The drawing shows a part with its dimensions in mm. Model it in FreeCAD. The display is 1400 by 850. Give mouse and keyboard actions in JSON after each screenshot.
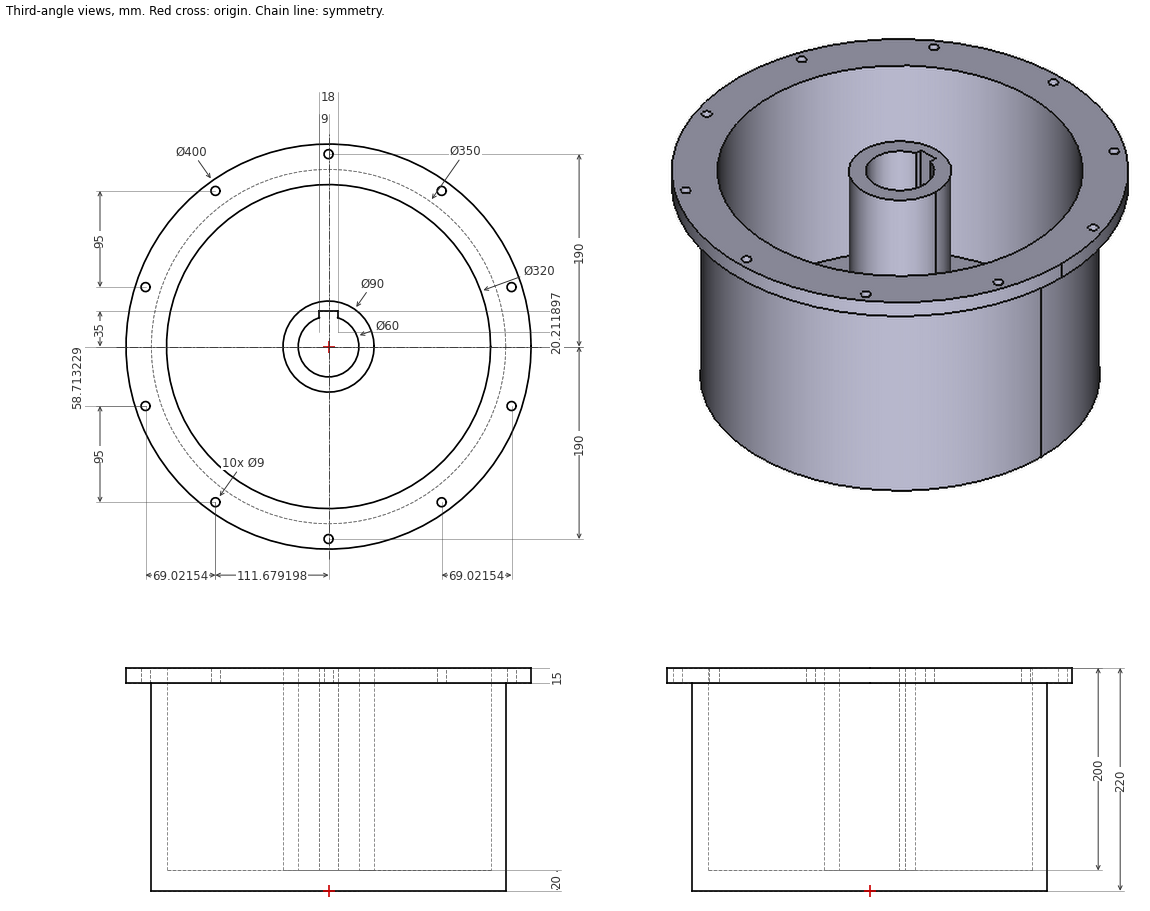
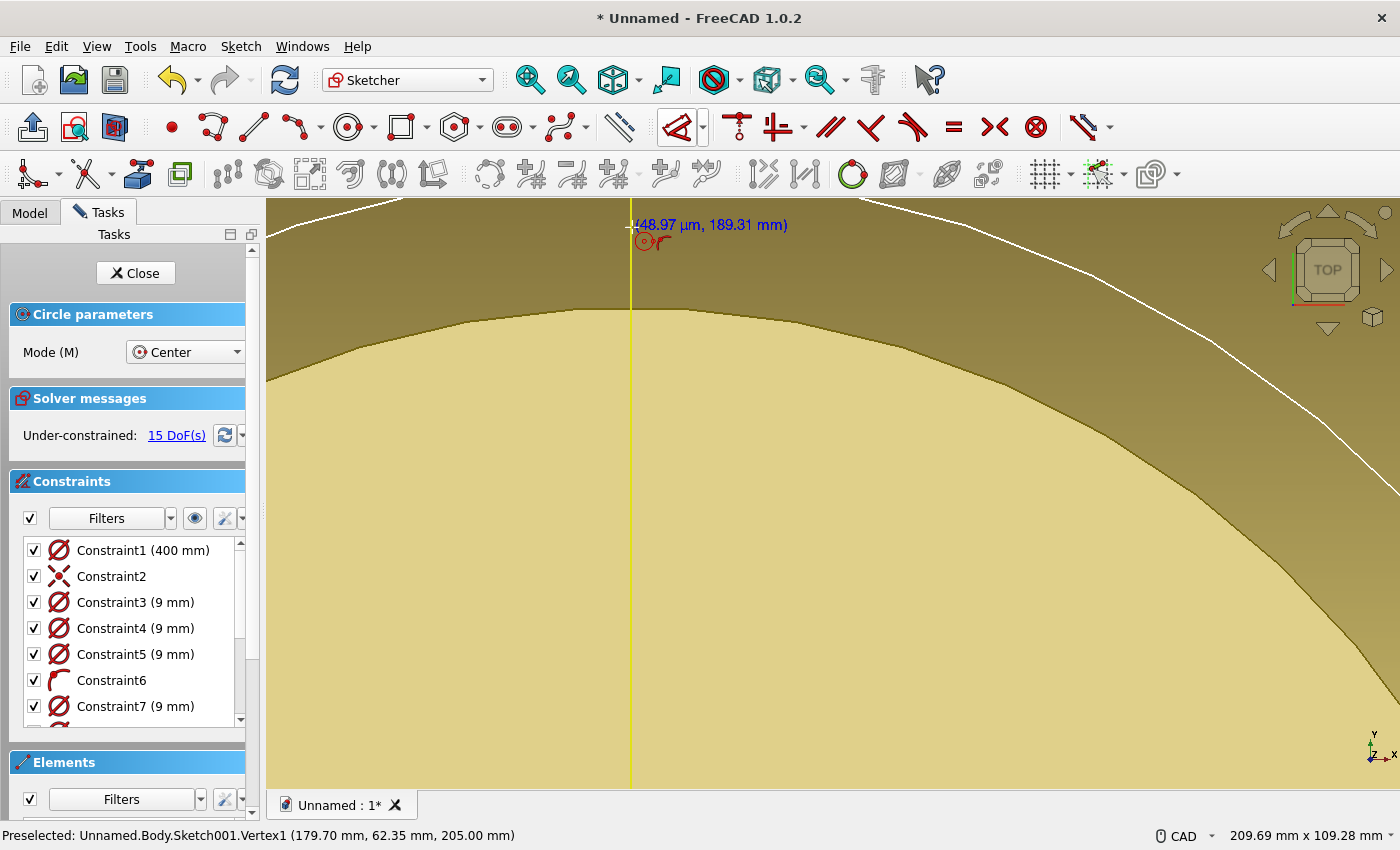
{"action": "scroll", "coordinate": [791, 343], "scroll_direction": "down", "scroll_amount": 9}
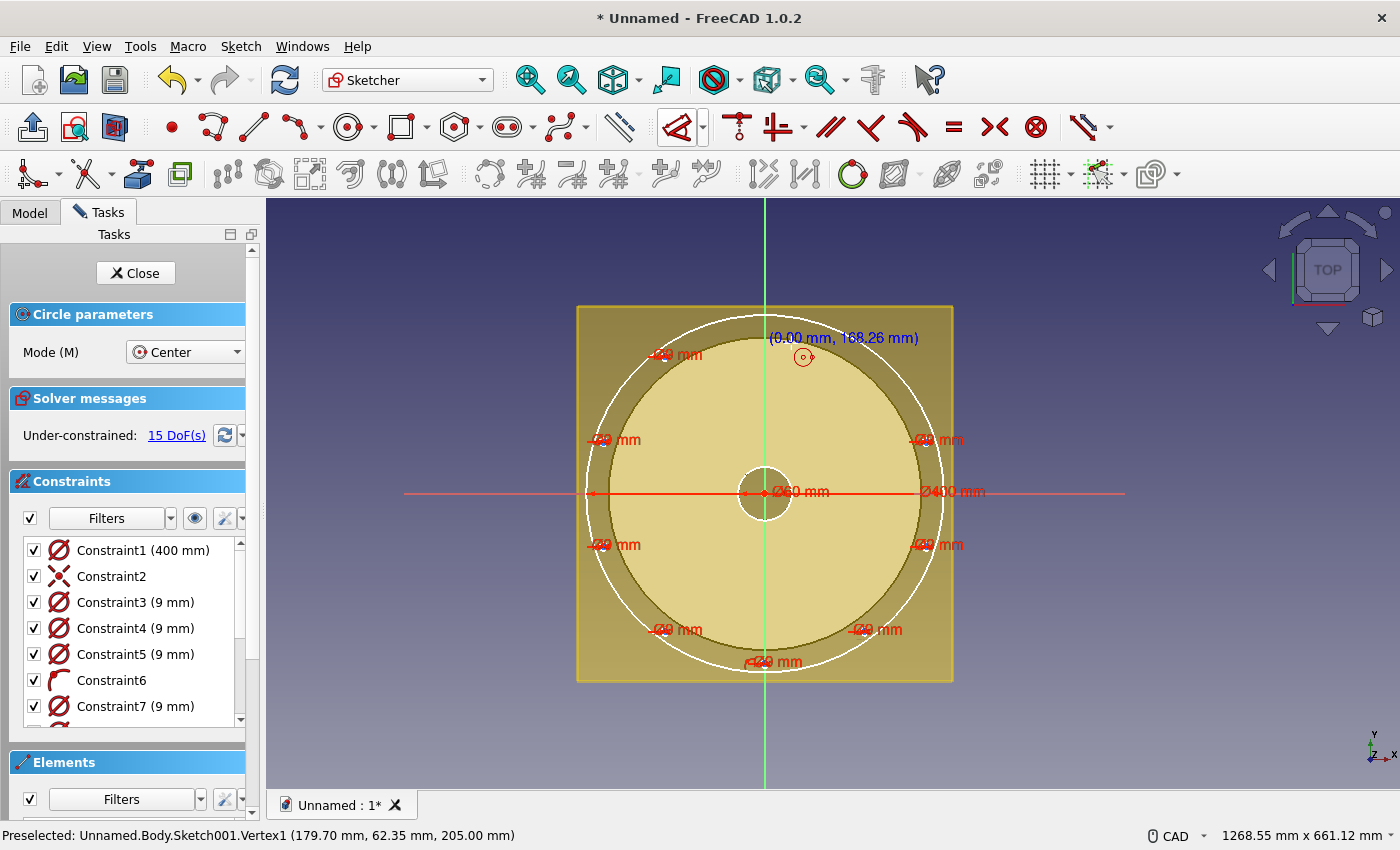
{"action": "scroll", "coordinate": [765, 324], "scroll_direction": "up", "scroll_amount": 3}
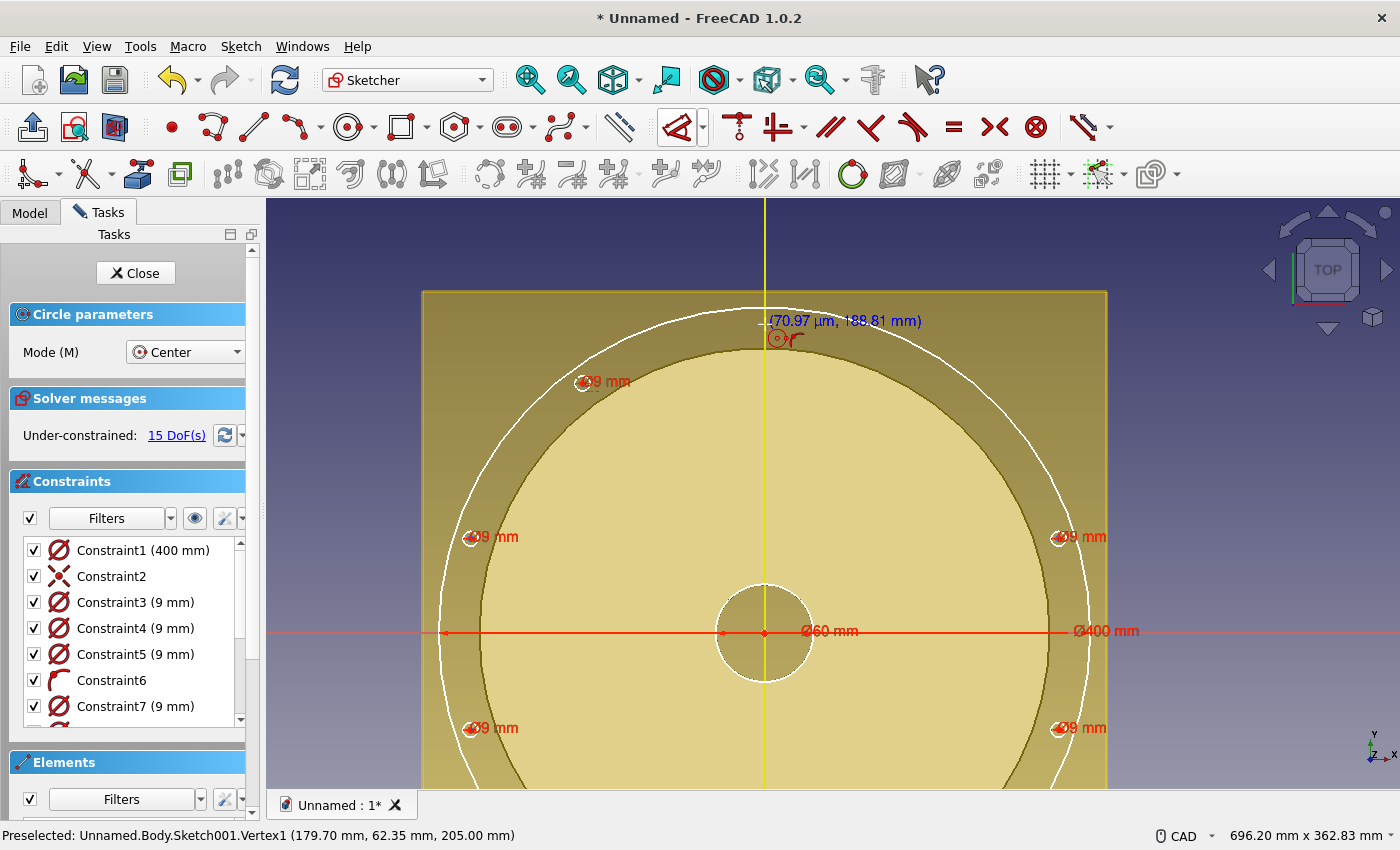
{"action": "left_click", "coordinate": [765, 324]}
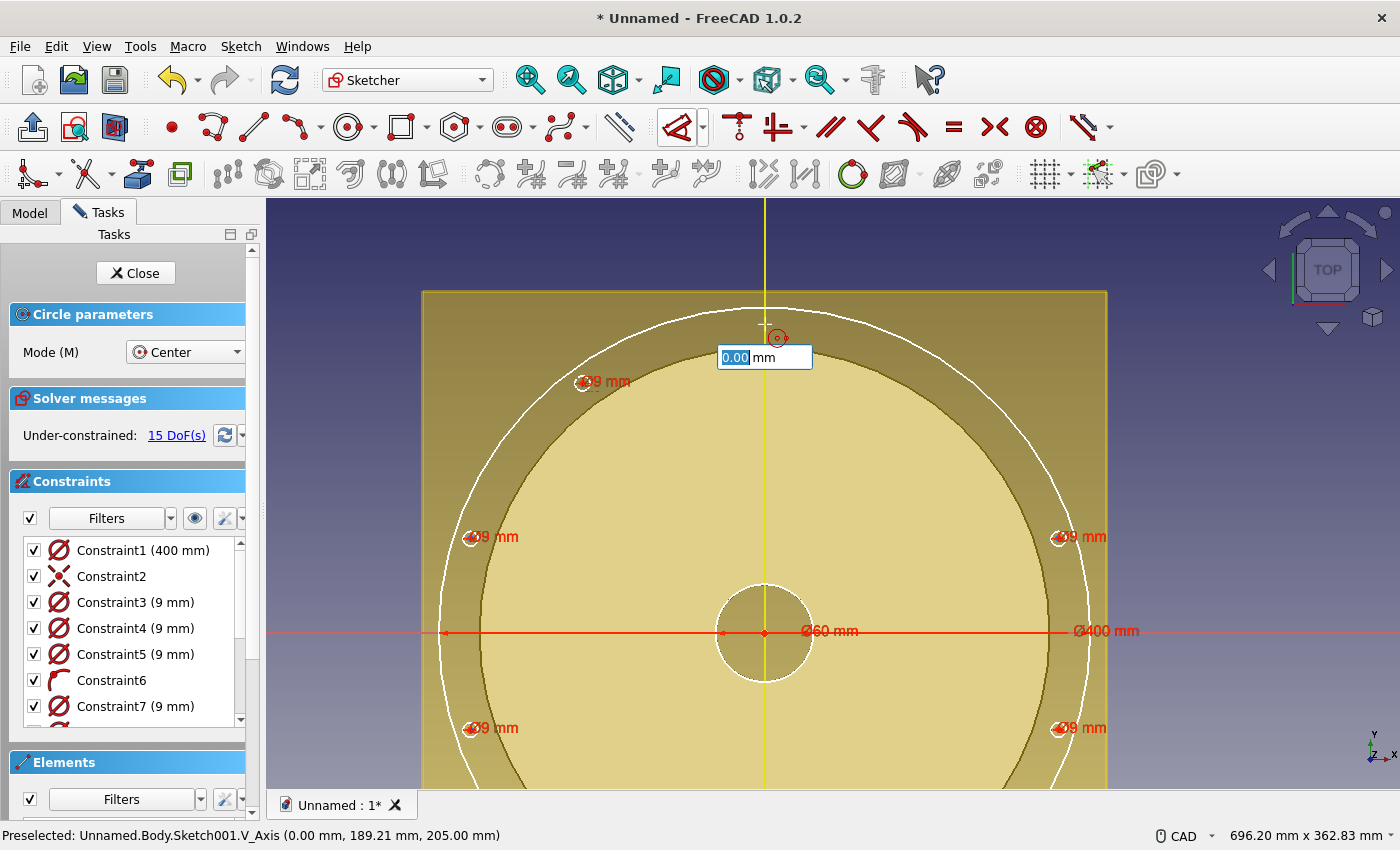
{"action": "scroll", "coordinate": [771, 321], "scroll_direction": "up", "scroll_amount": 5}
{"action": "mouse_move", "coordinate": [771, 321]}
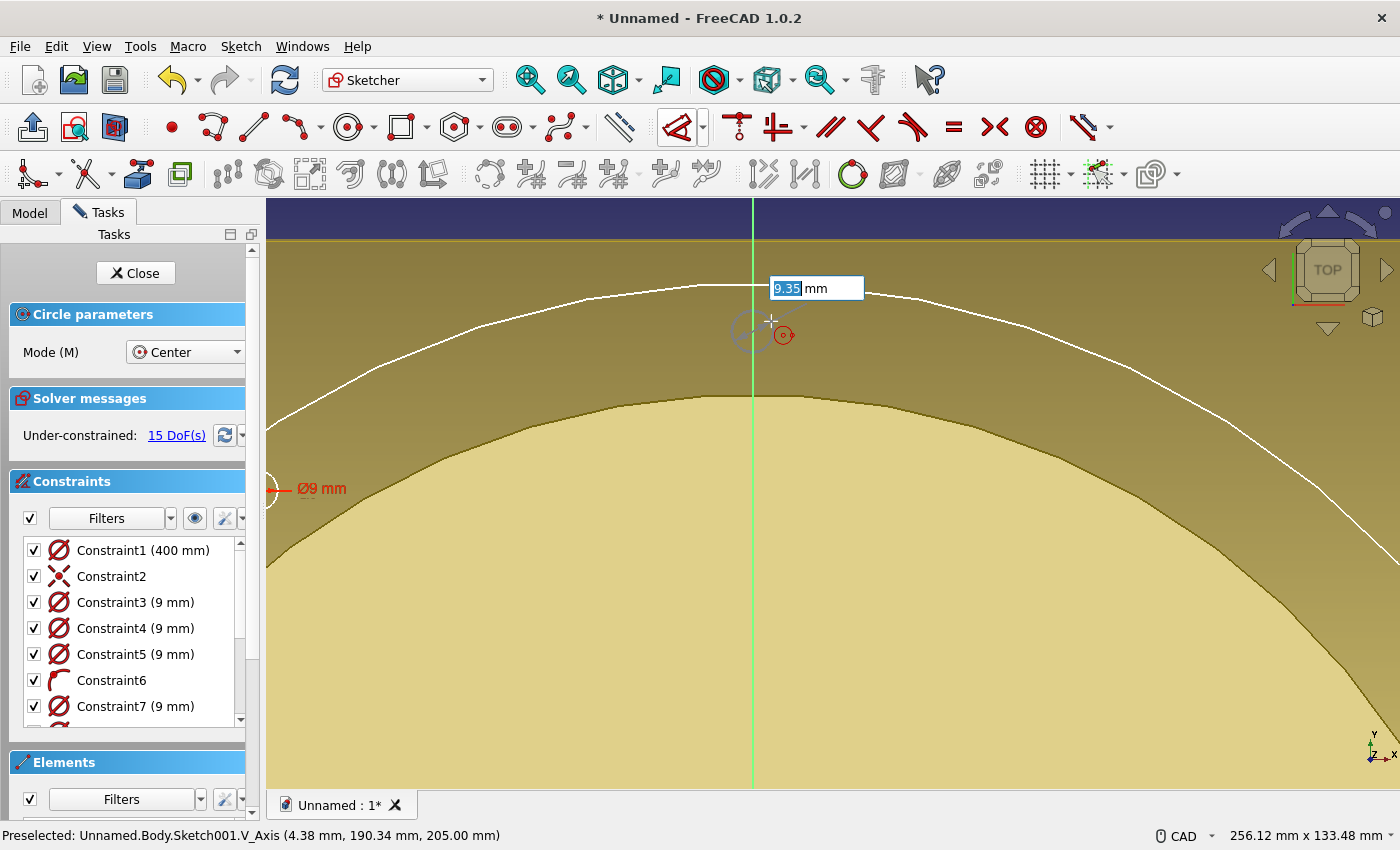
{"action": "type", "text": "9"}
{"action": "key", "text": "Return"}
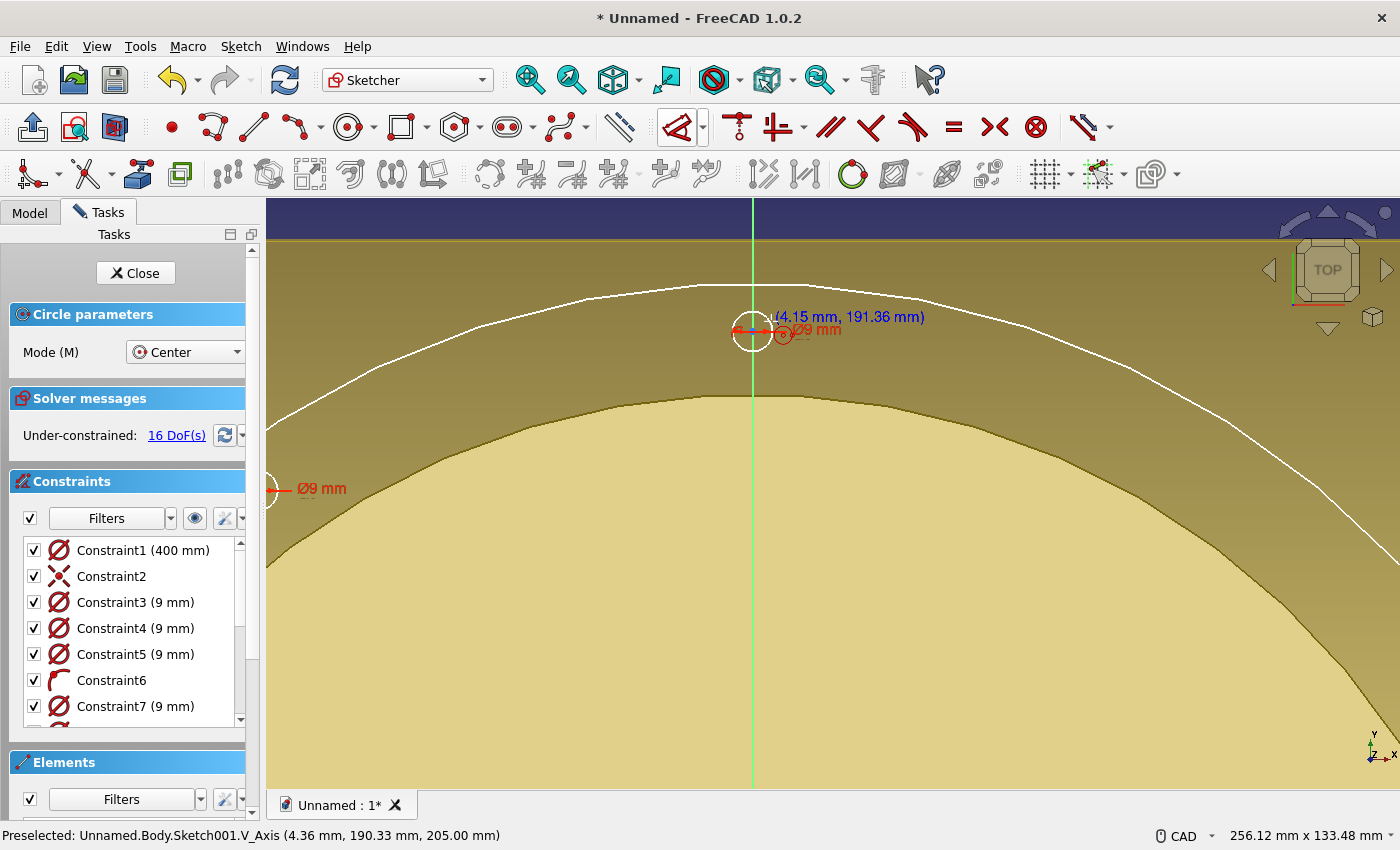
{"action": "scroll", "coordinate": [768, 323], "scroll_direction": "down", "scroll_amount": 8}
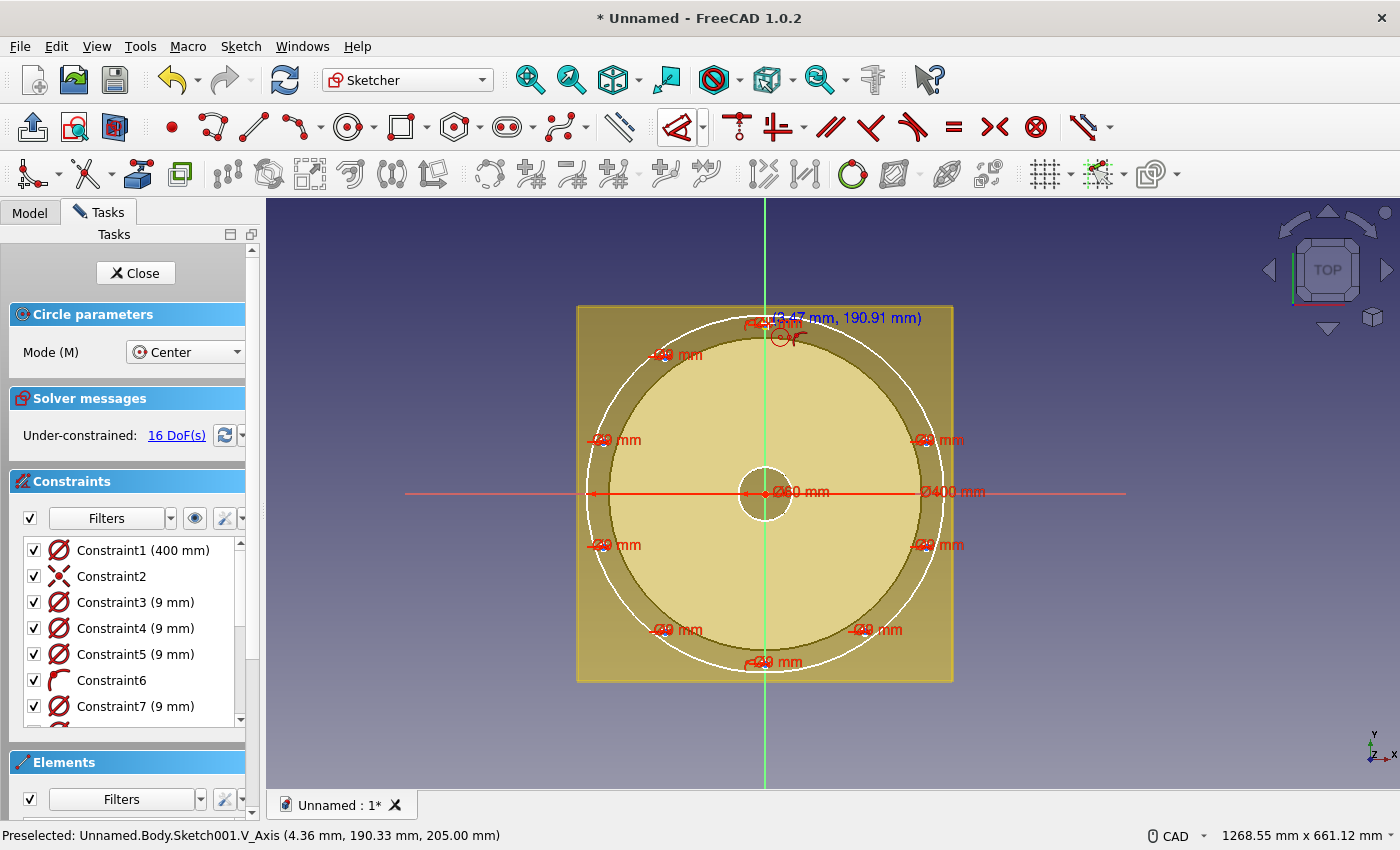
{"action": "scroll", "coordinate": [865, 357], "scroll_direction": "up", "scroll_amount": 9}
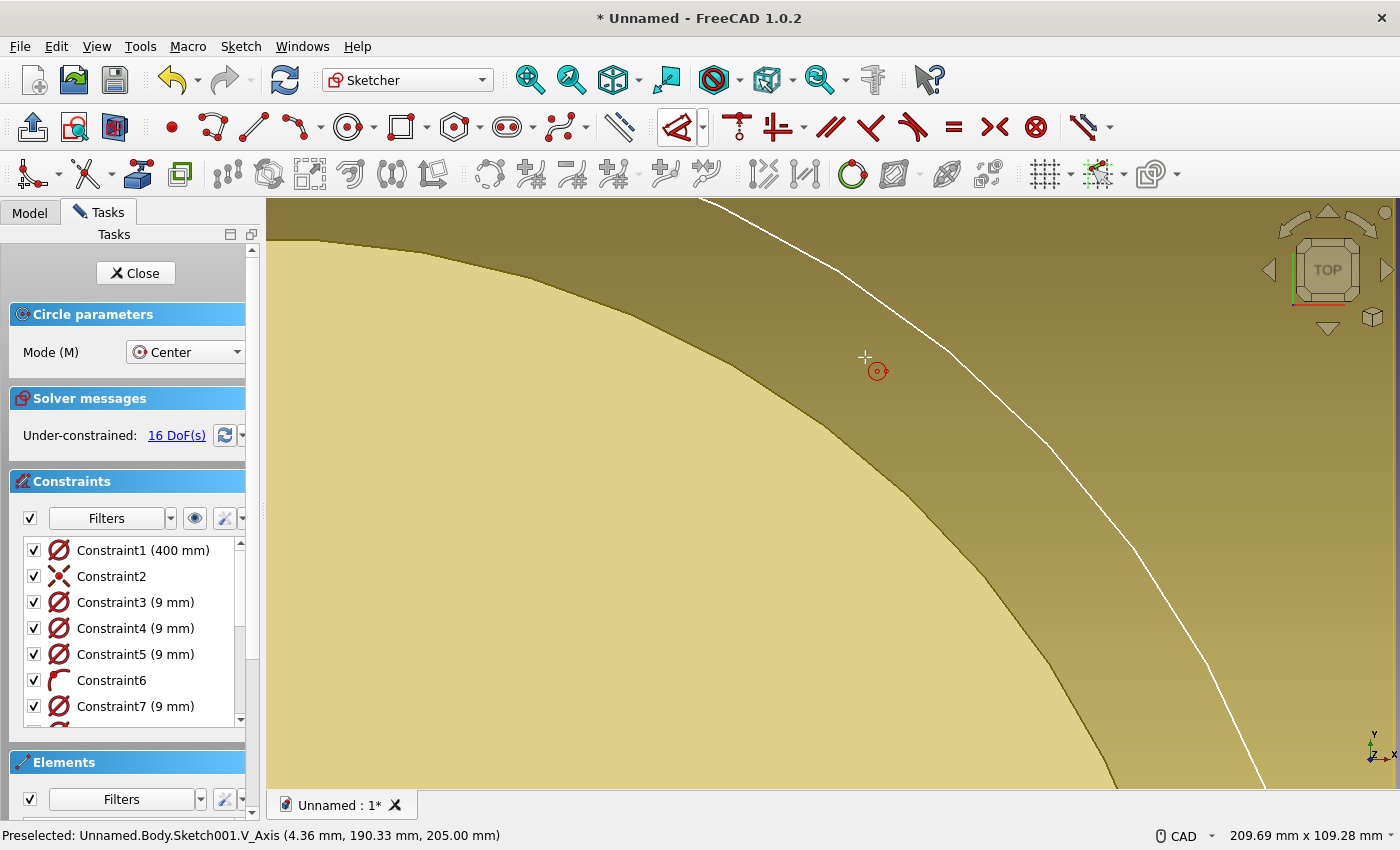
{"action": "scroll", "coordinate": [865, 357], "scroll_direction": "down", "scroll_amount": 9}